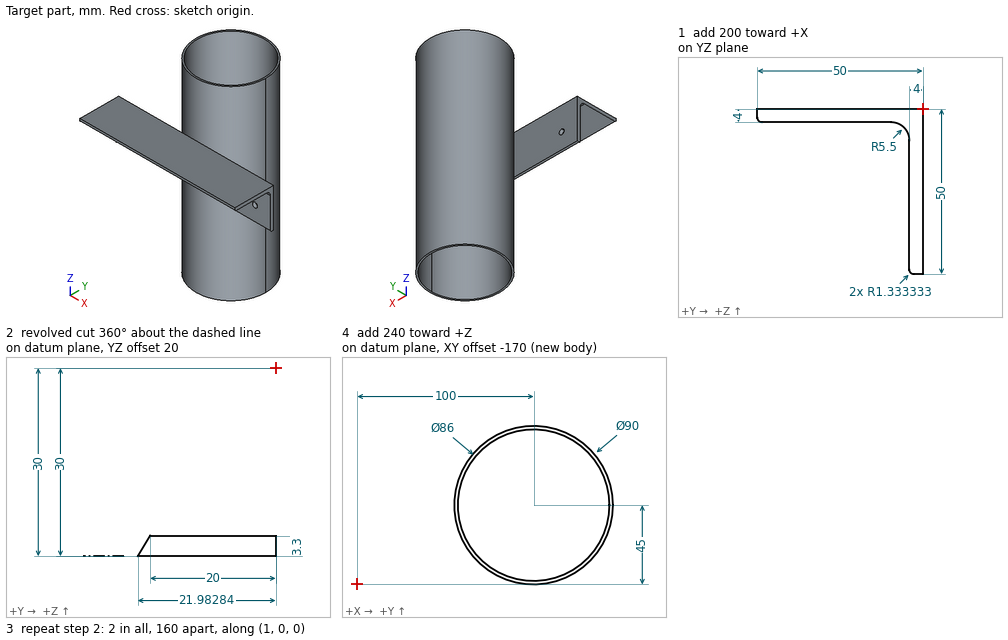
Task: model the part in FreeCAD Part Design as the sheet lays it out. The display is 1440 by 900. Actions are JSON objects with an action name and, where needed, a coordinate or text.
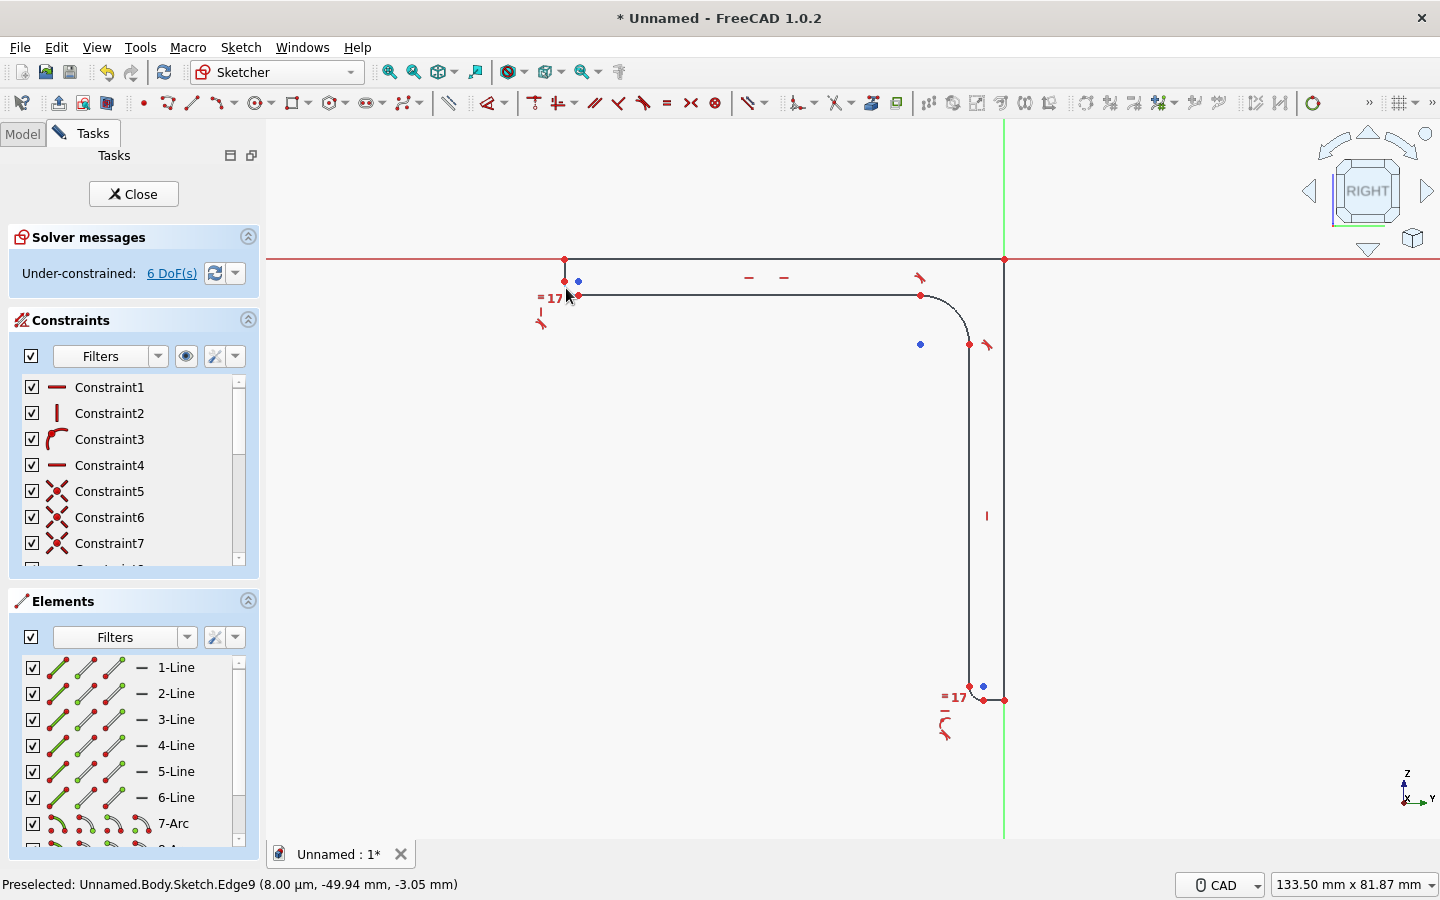
{"action": "left_click", "coordinate": [964, 322]}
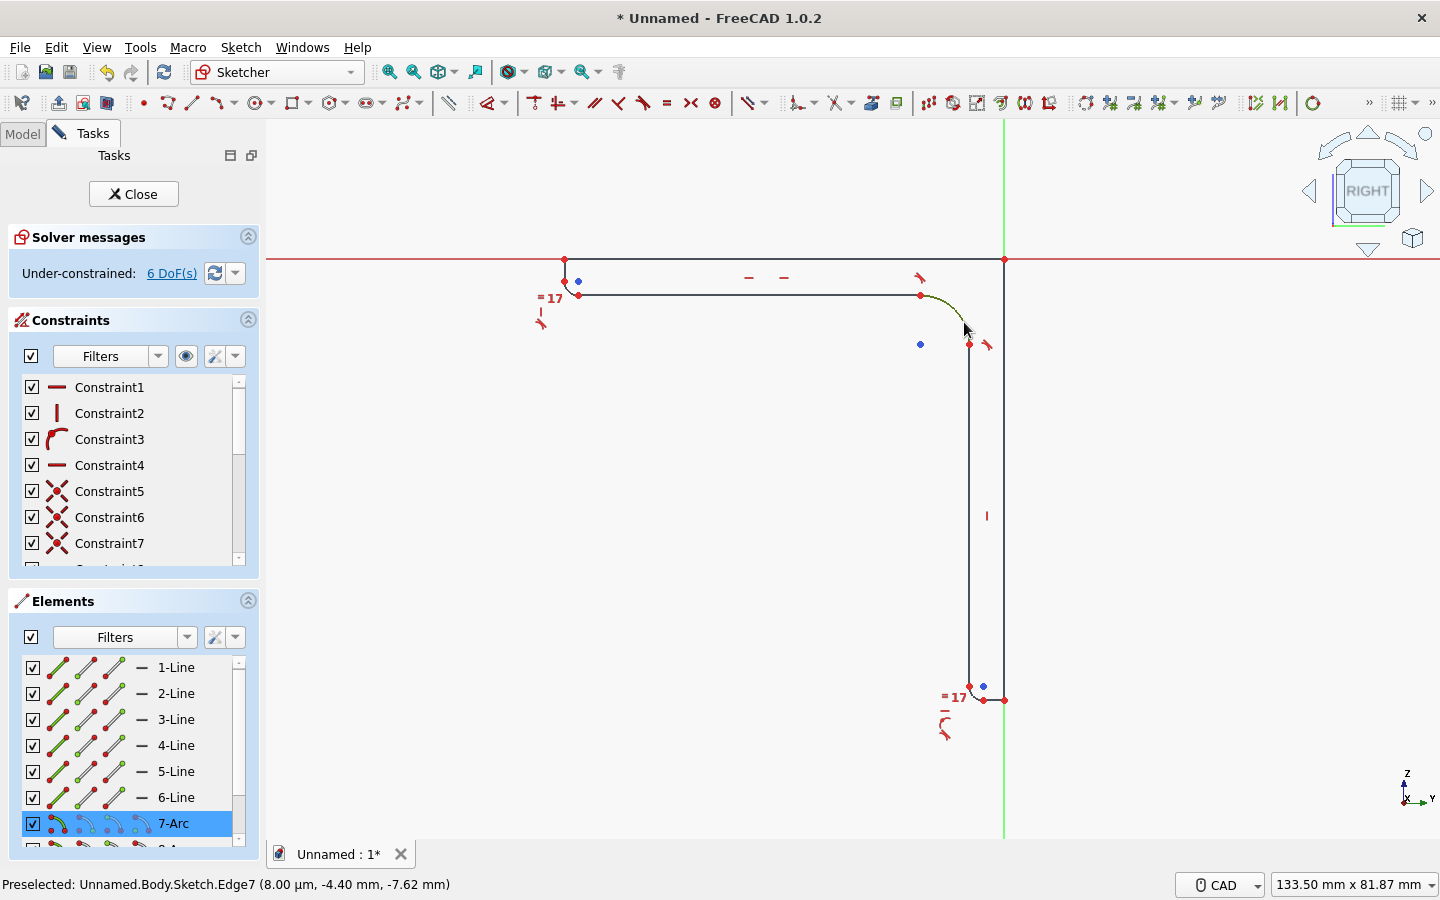
{"action": "key", "text": "k r"}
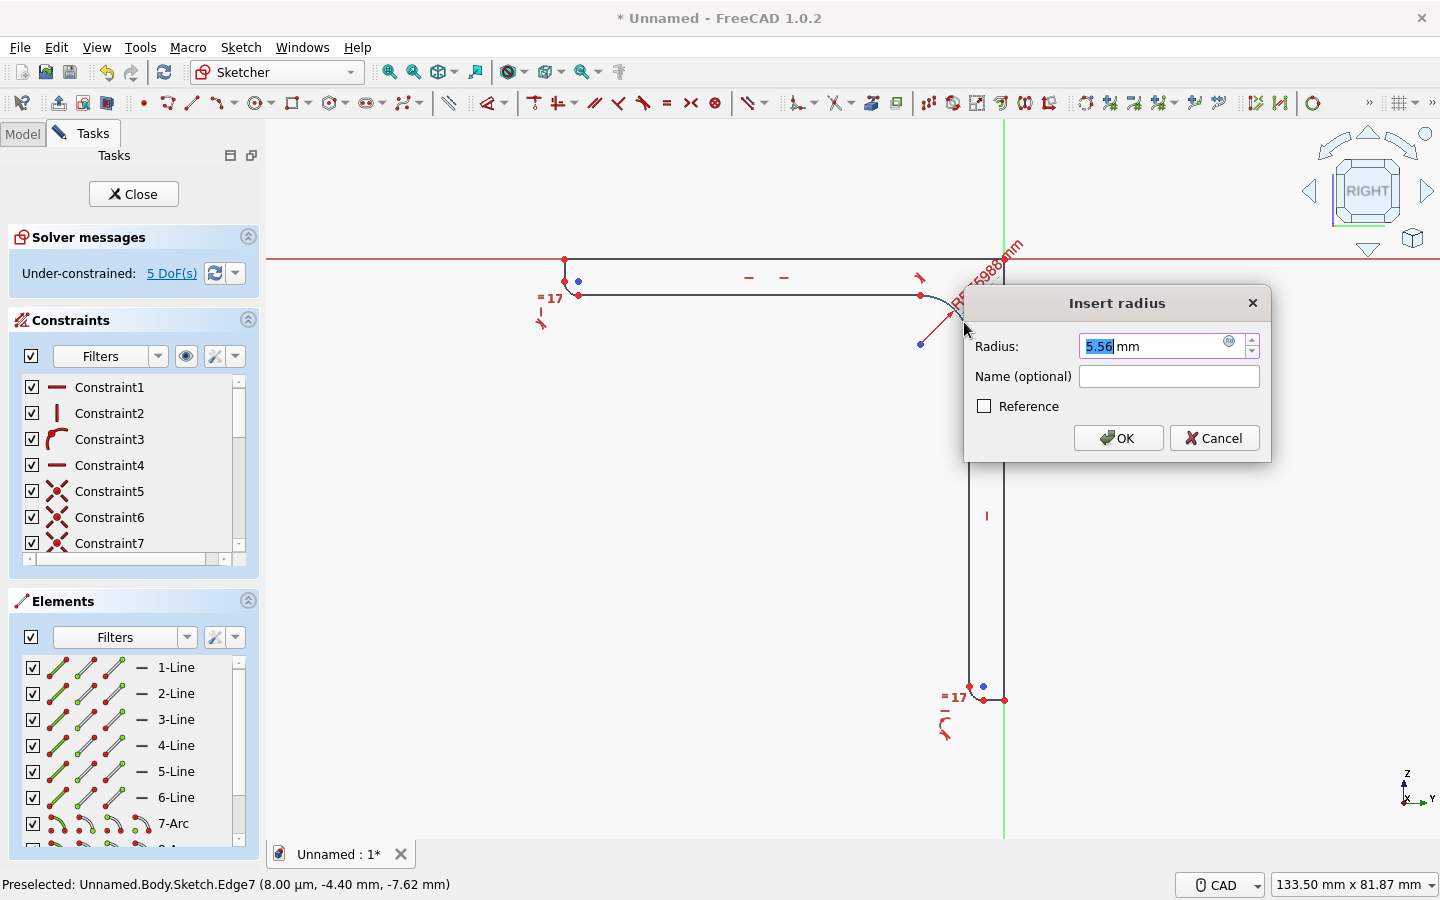
{"action": "type", "text": "5.5"}
{"action": "key", "text": "Return"}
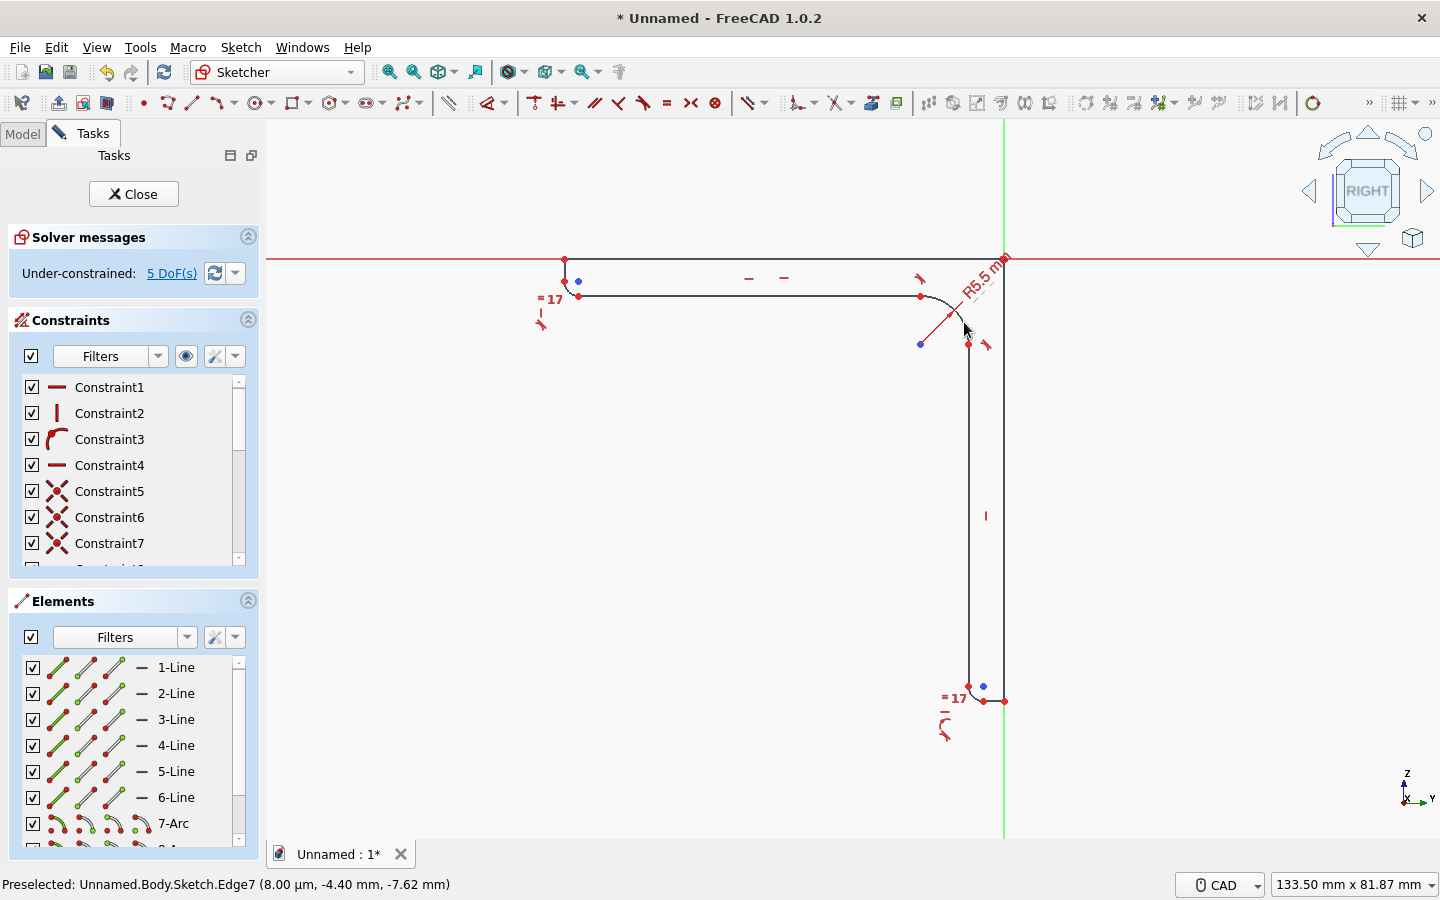
{"action": "scroll", "coordinate": [973, 697], "scroll_direction": "up", "scroll_amount": 7}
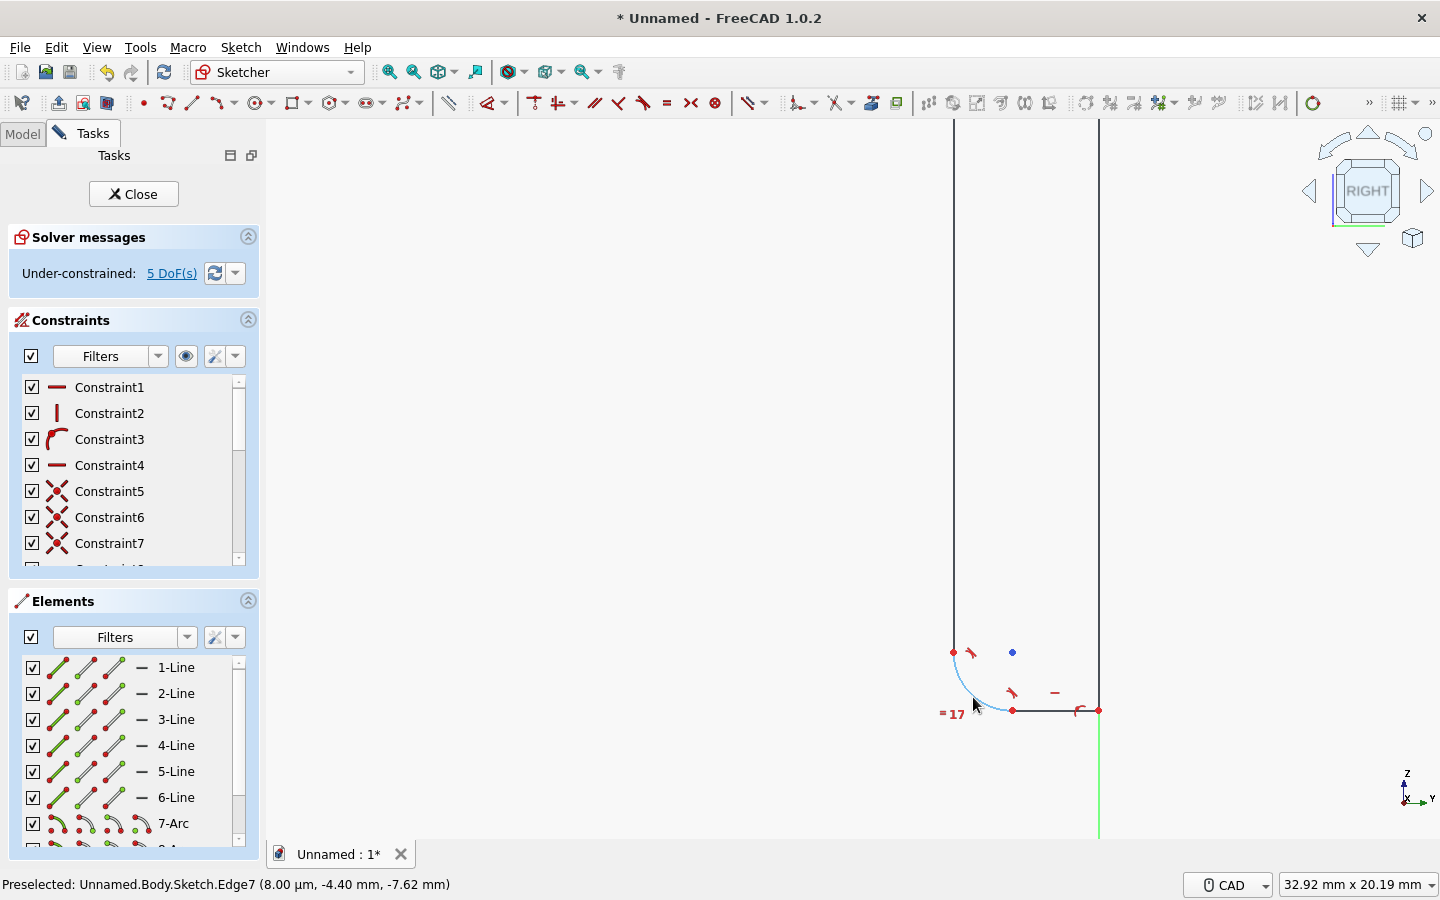
{"action": "left_click", "coordinate": [971, 694]}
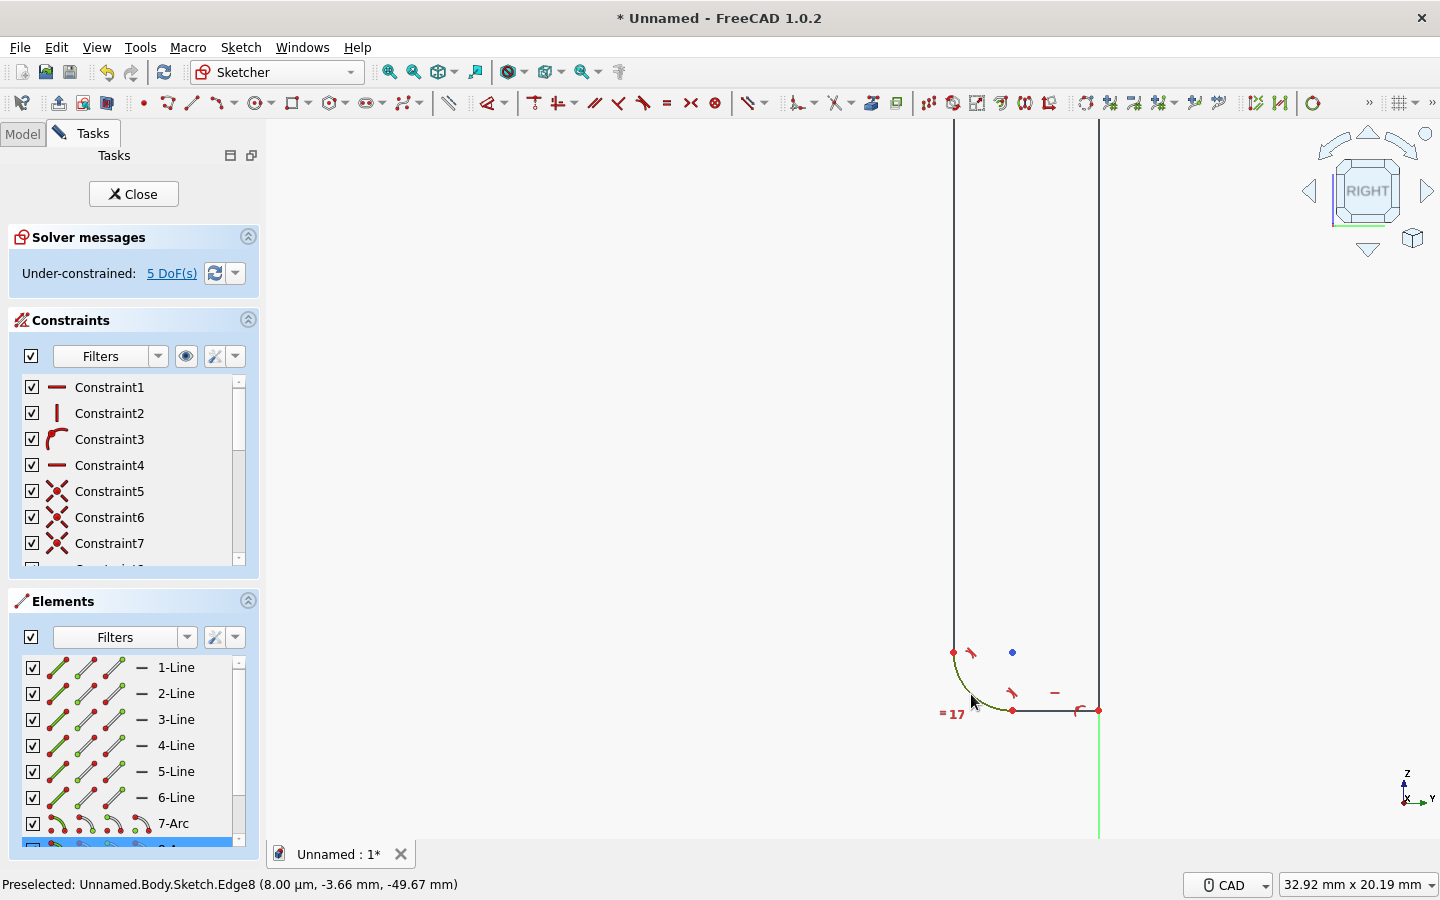
{"action": "key", "text": "k r"}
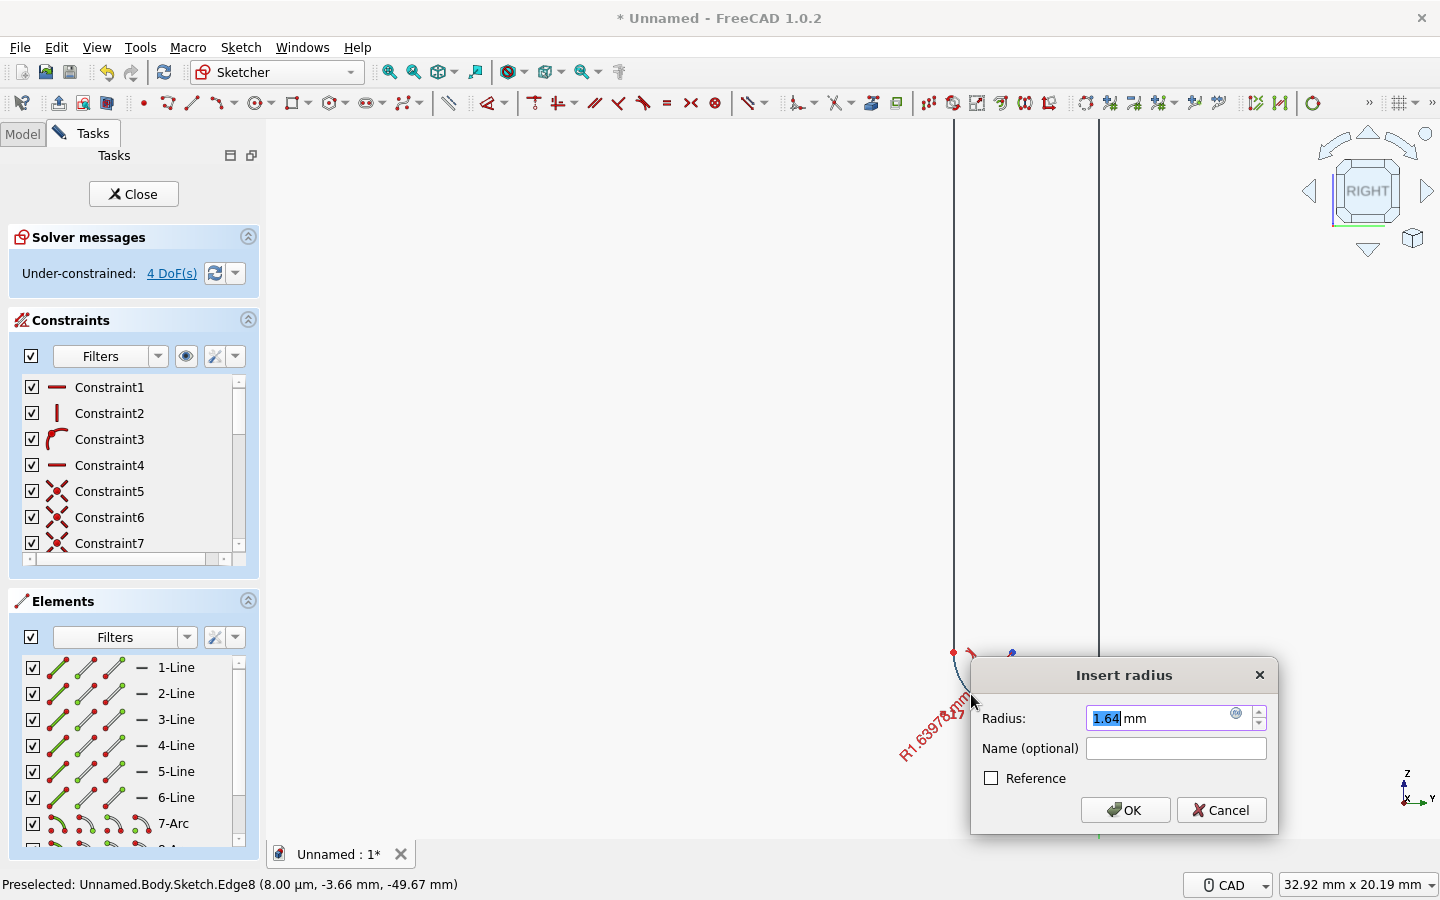
{"action": "type", "text": "1.333333"}
{"action": "key", "text": "Return"}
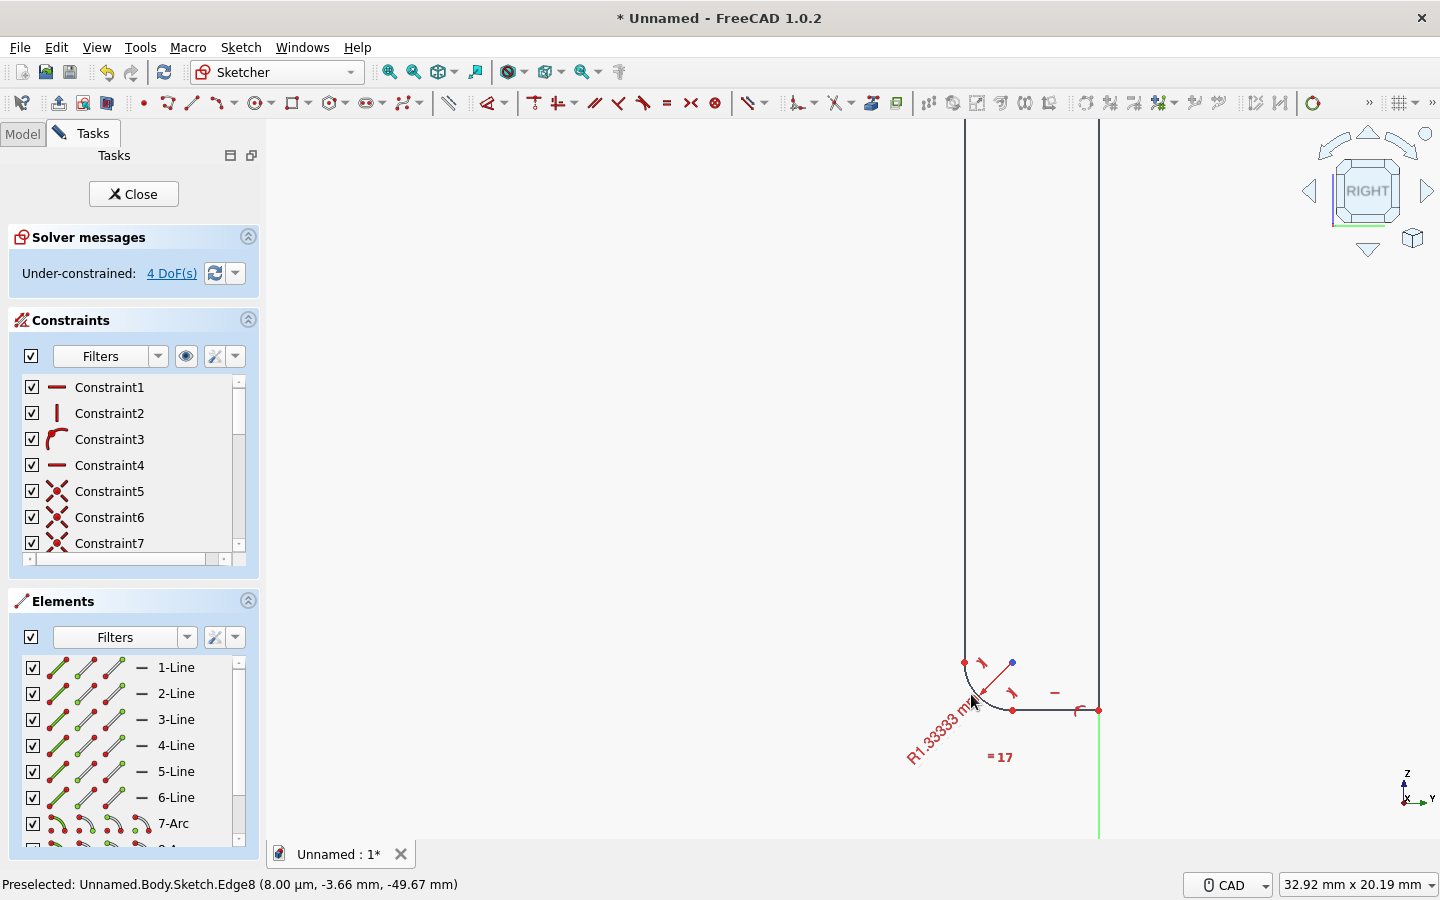
{"action": "scroll", "coordinate": [973, 698], "scroll_direction": "down", "scroll_amount": 7}